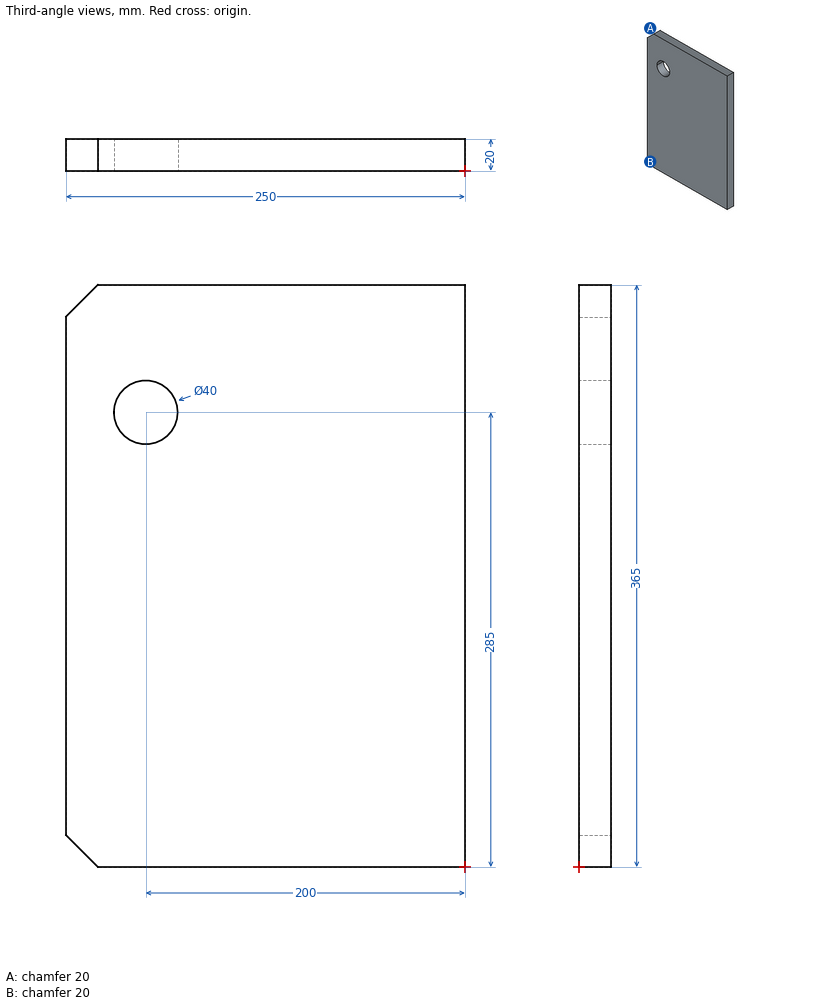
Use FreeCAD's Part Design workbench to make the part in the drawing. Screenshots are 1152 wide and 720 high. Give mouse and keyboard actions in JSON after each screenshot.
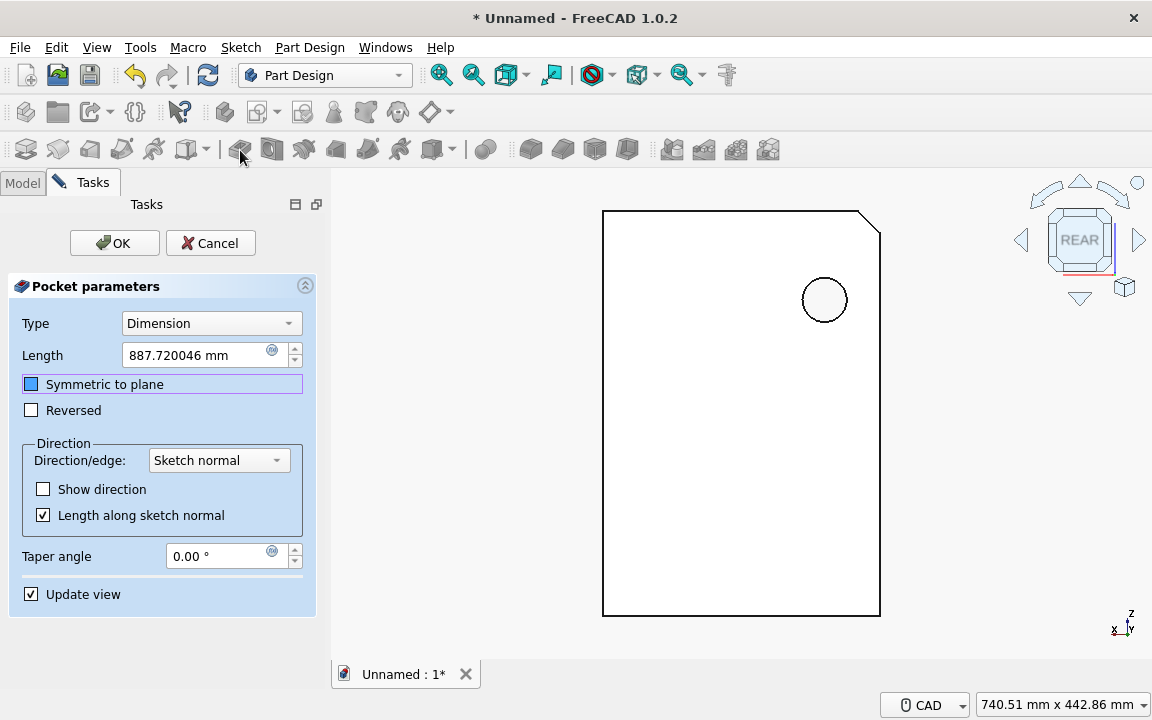
{"action": "left_click", "coordinate": [30, 384]}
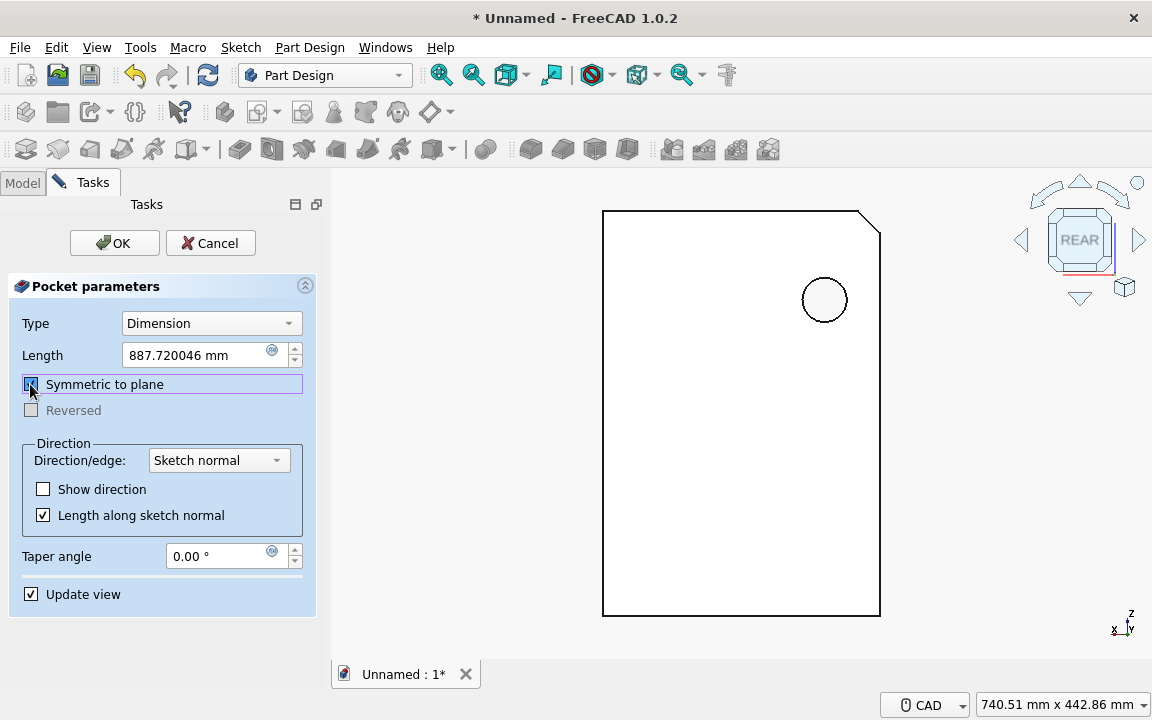
{"action": "left_click", "coordinate": [115, 243]}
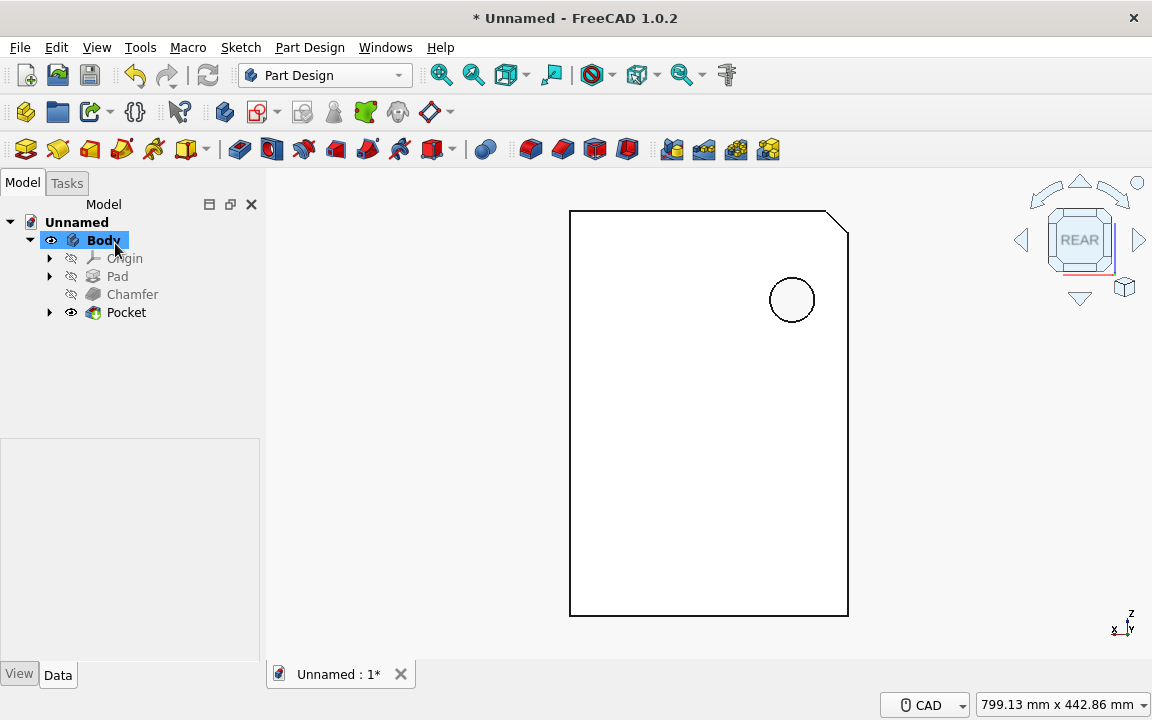
{"action": "key", "text": "0"}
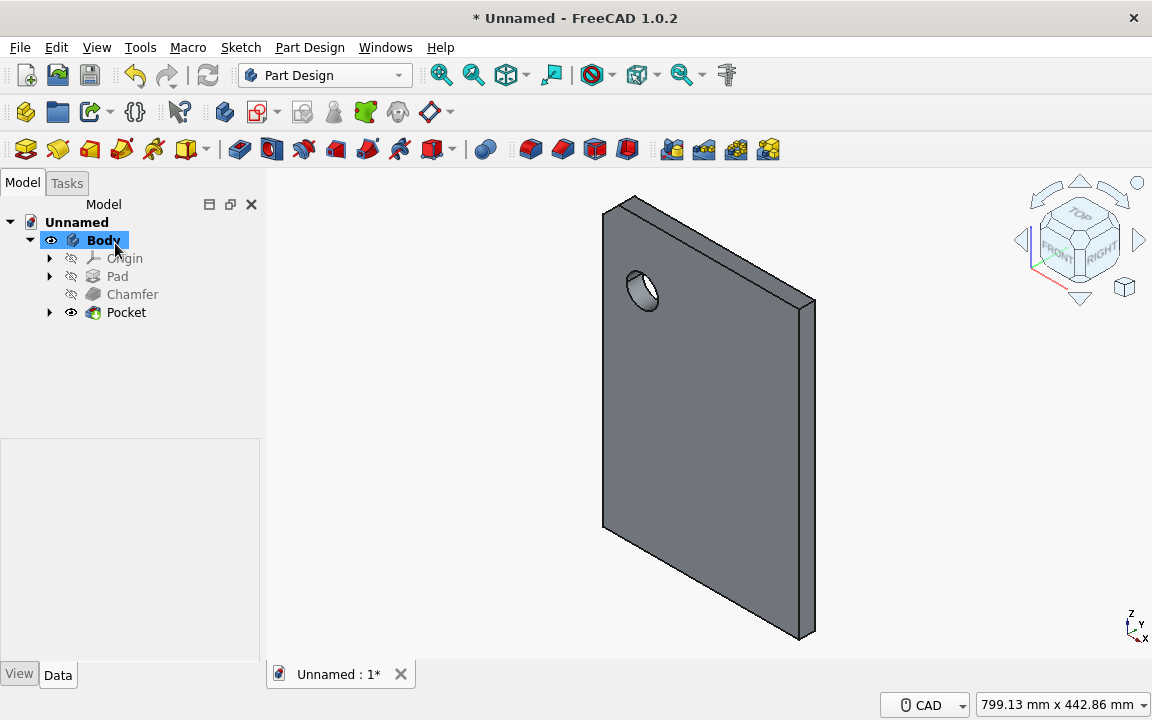
{"action": "key", "text": "2"}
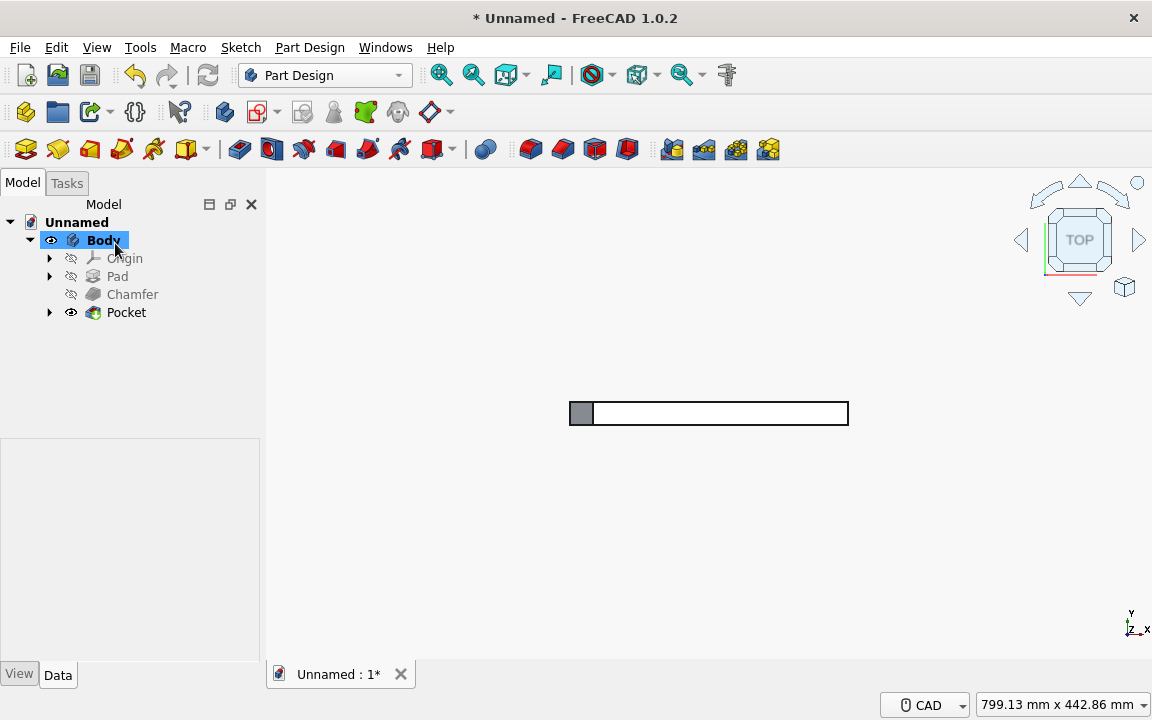
{"action": "key", "text": "v f"}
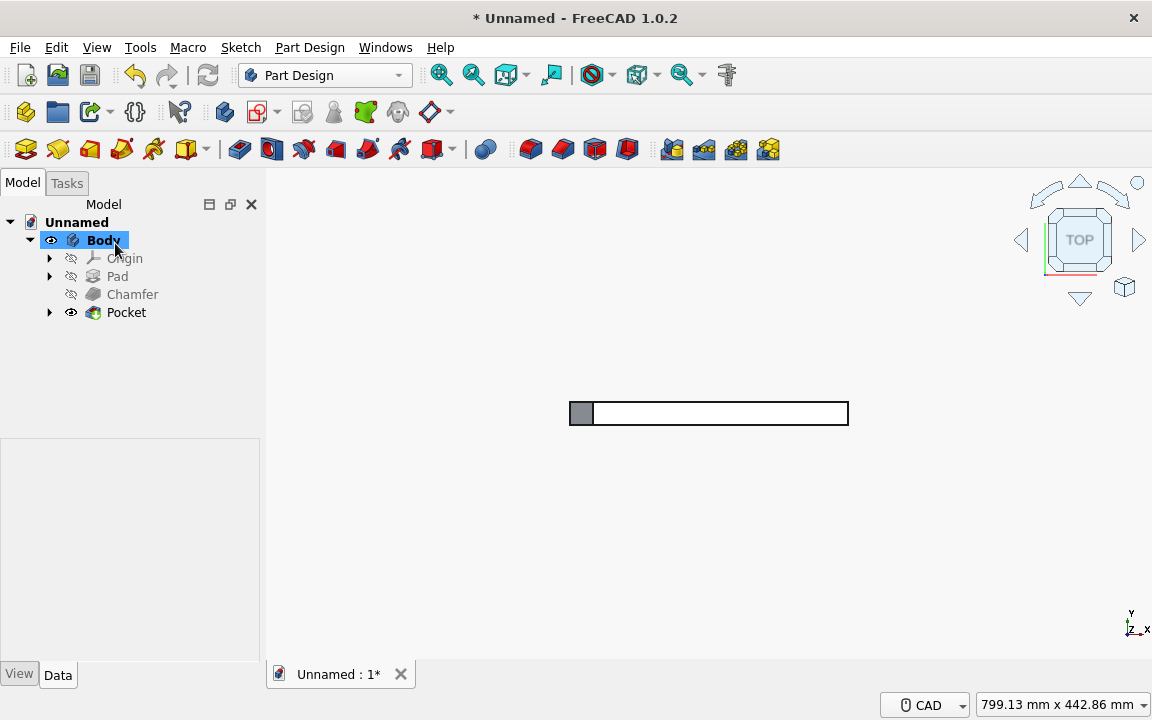
{"action": "key", "text": "1"}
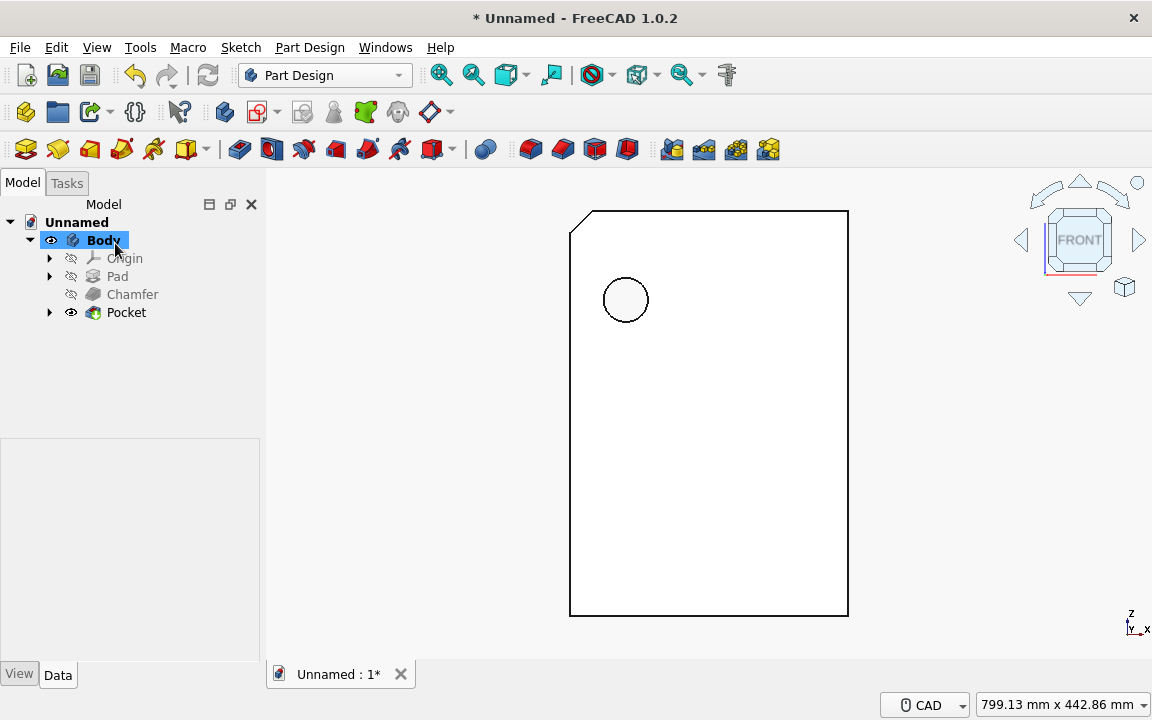
{"action": "key", "text": "3"}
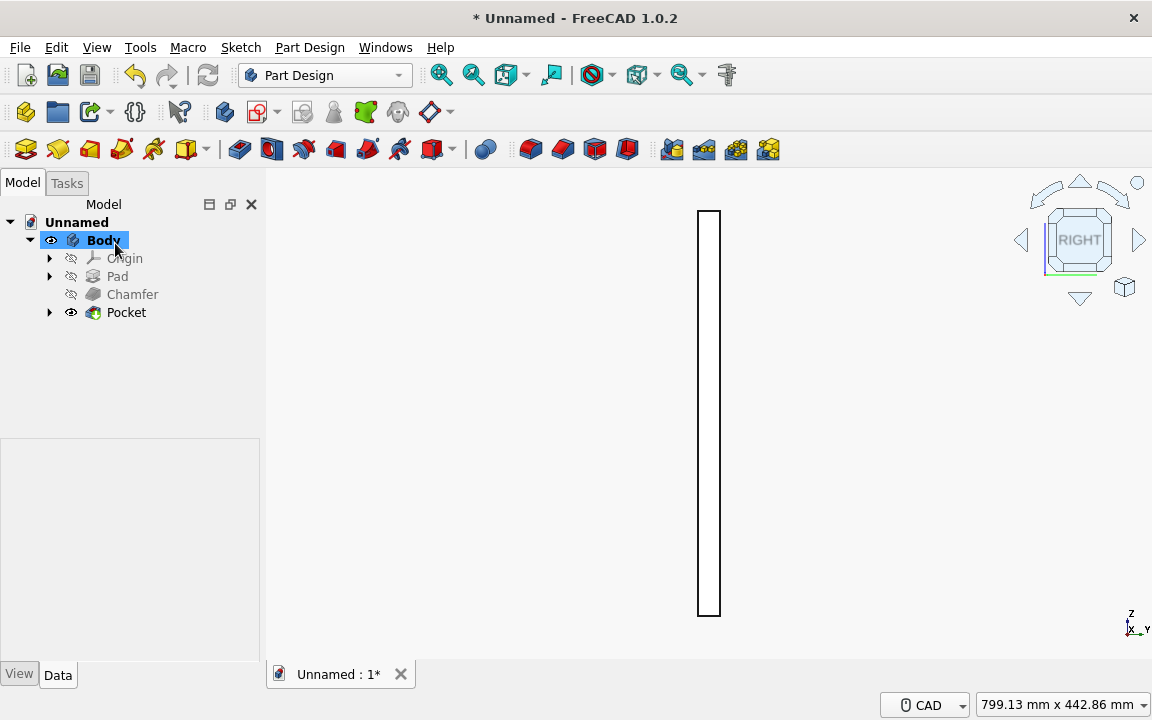
{"action": "key", "text": "5"}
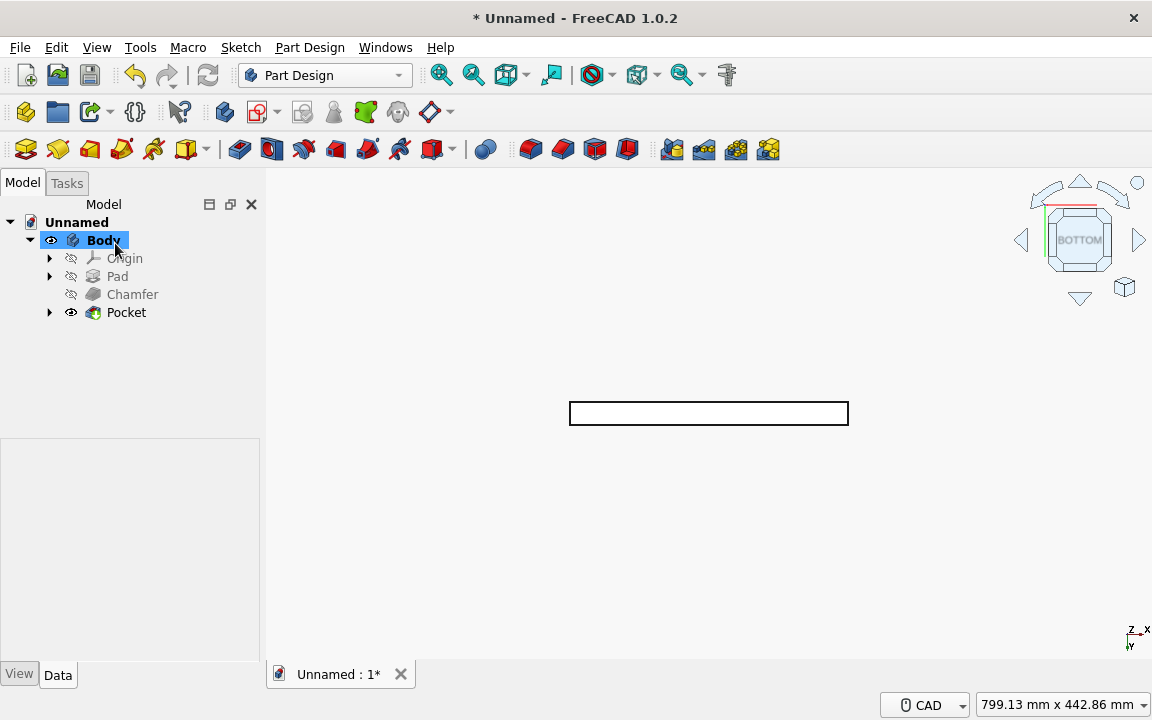
{"action": "key", "text": "v f"}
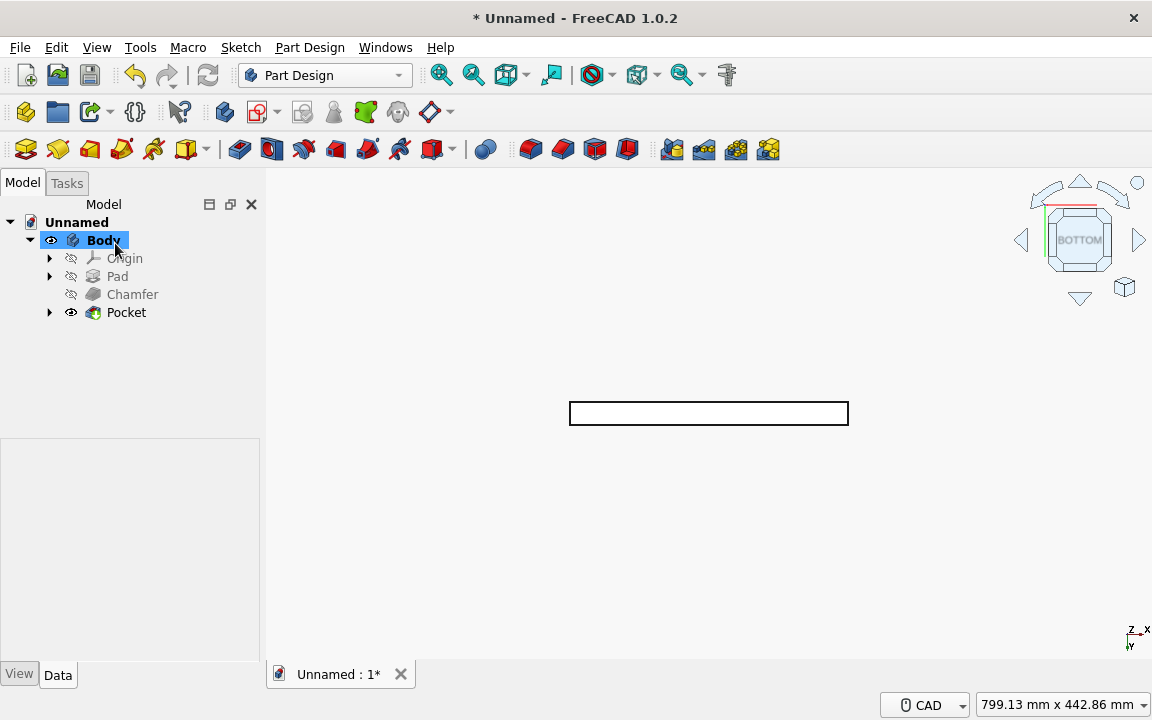
{"action": "left_click", "coordinate": [570, 412]}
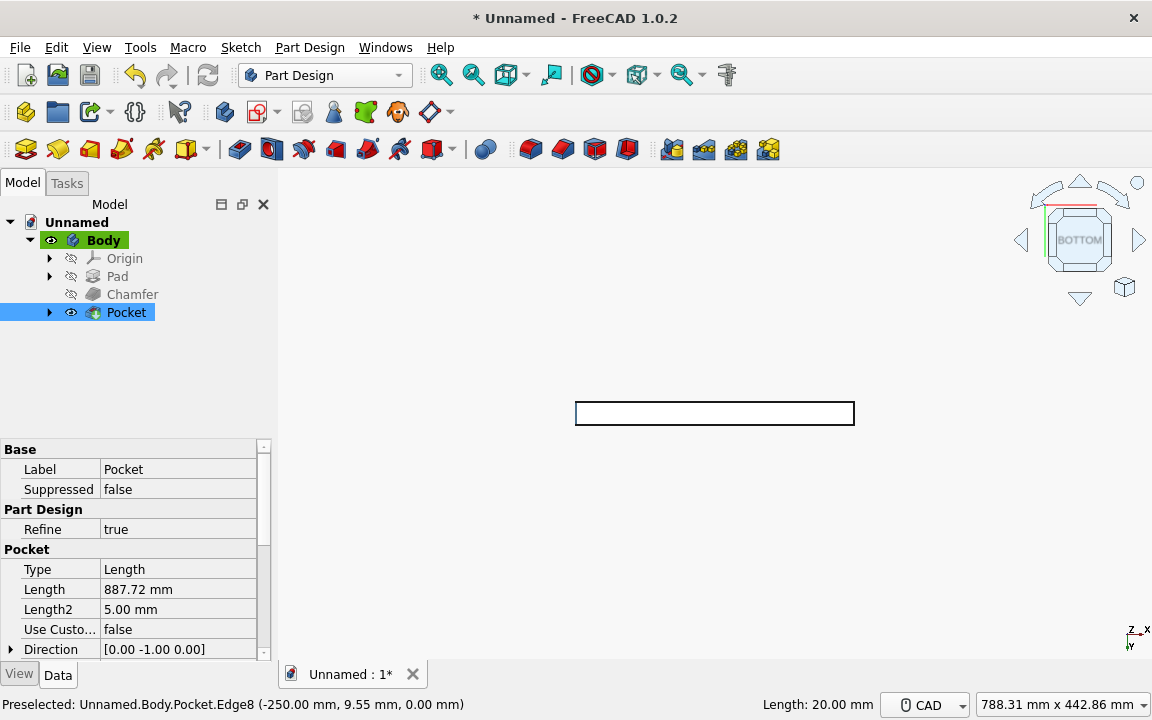
{"action": "left_click", "coordinate": [564, 150]}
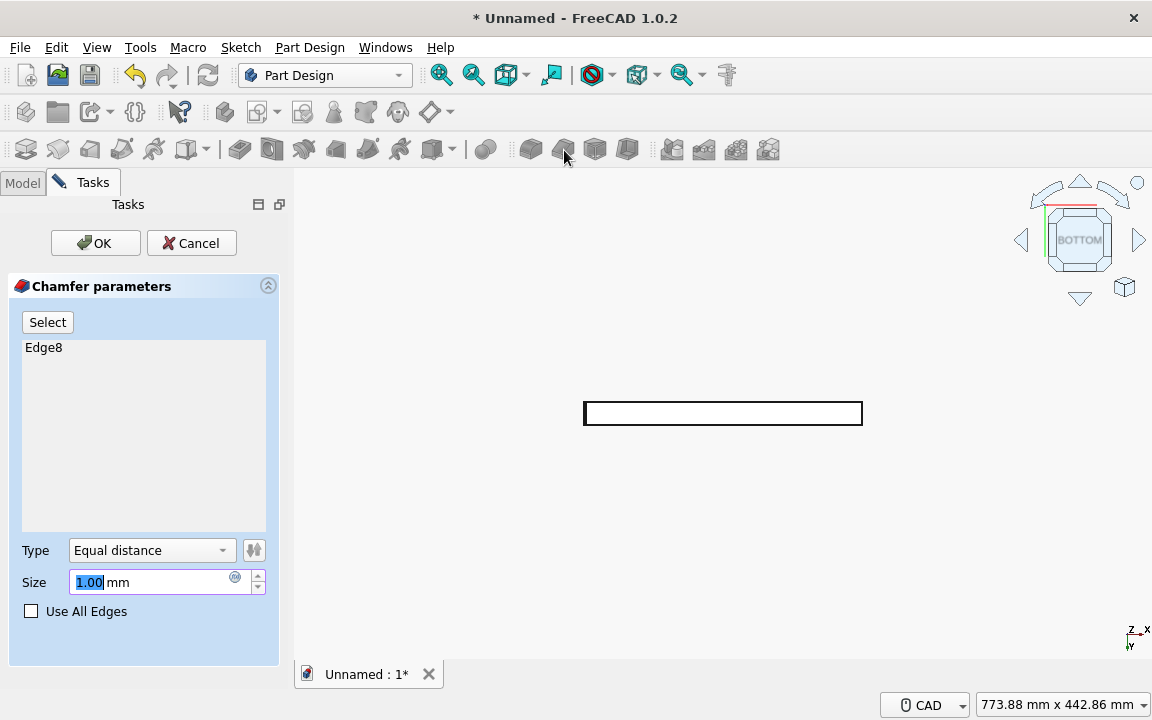
{"action": "type", "text": "20"}
{"action": "key", "text": "Tab"}